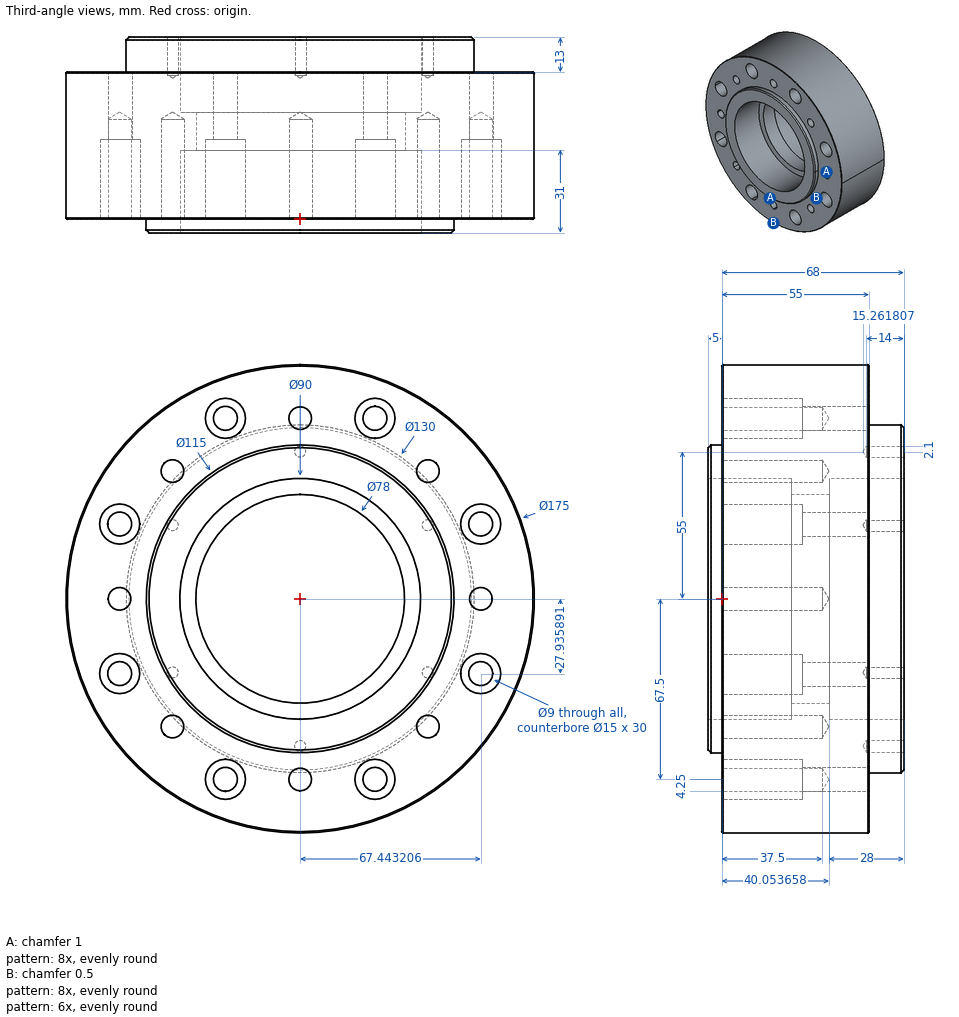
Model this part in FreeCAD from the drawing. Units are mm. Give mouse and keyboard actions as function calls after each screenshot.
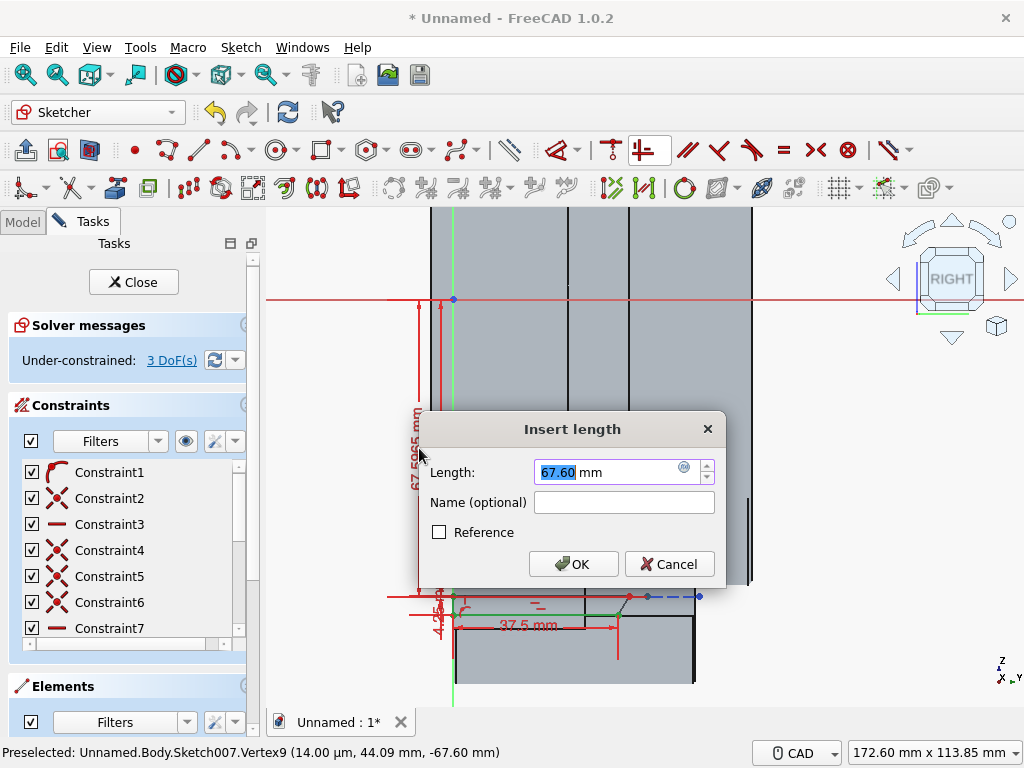
text(67.5)
key(Return)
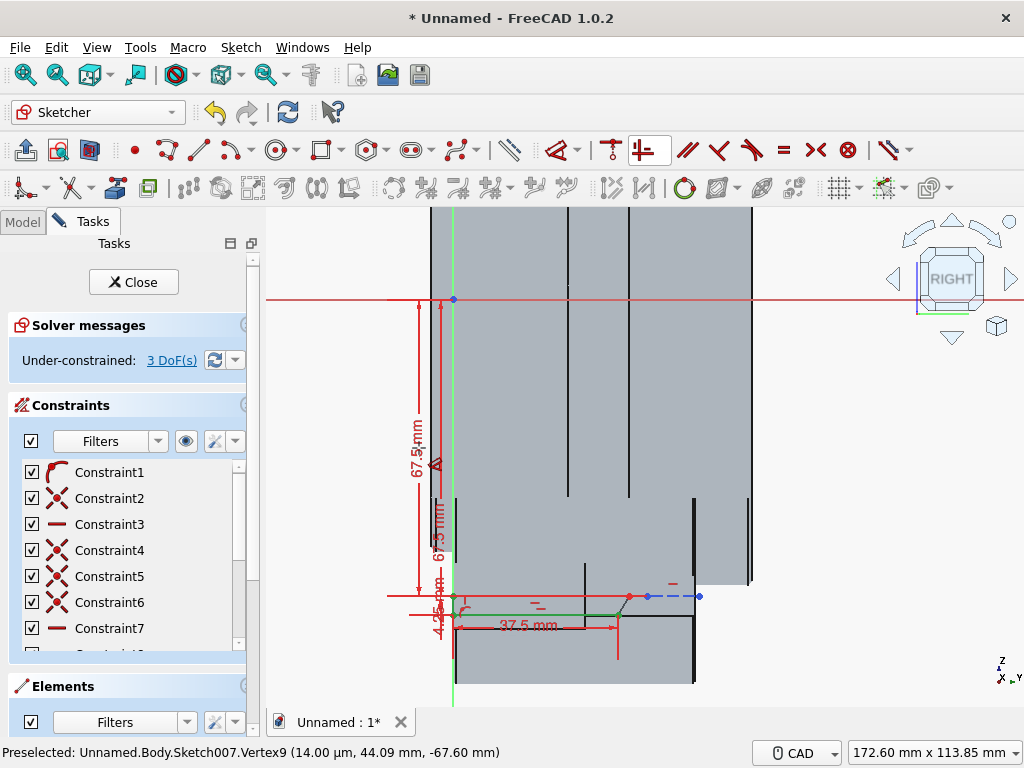
click(576, 596)
click(603, 630)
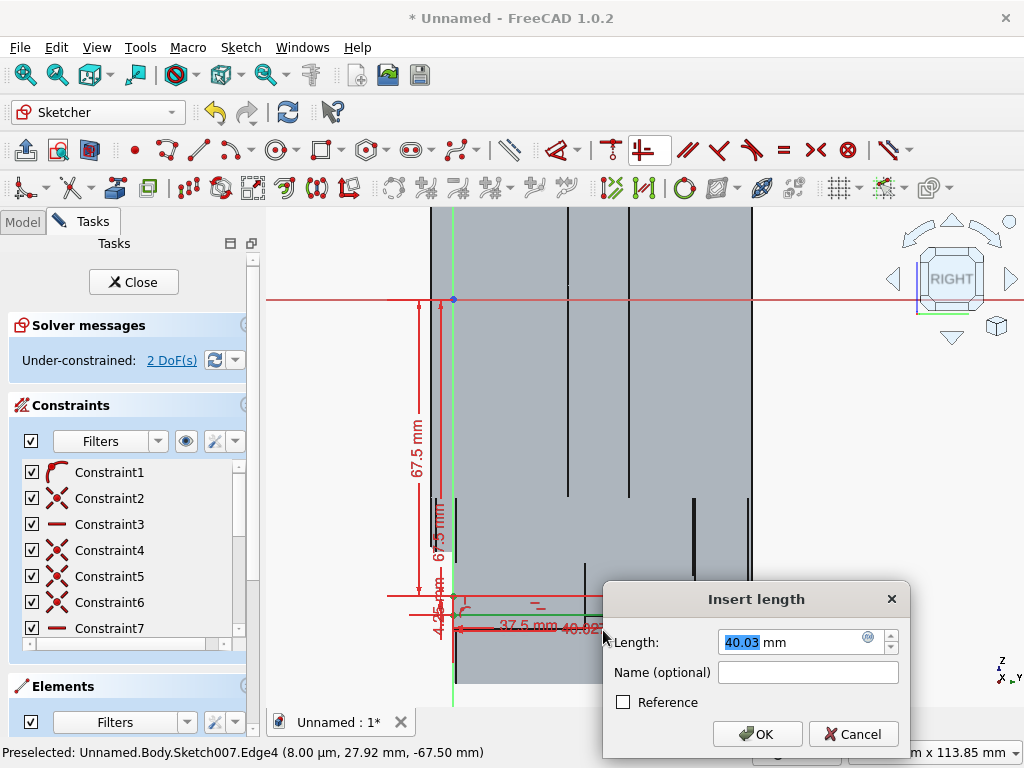
text(40.053658)
key(Return)
key(Escape)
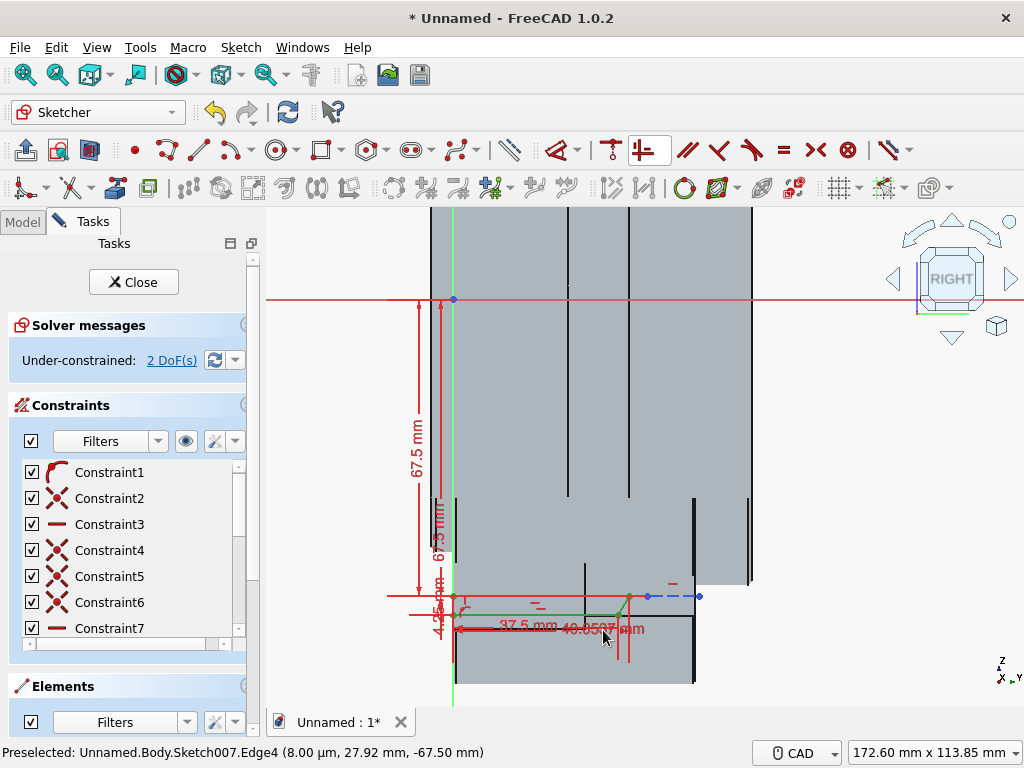
click(134, 282)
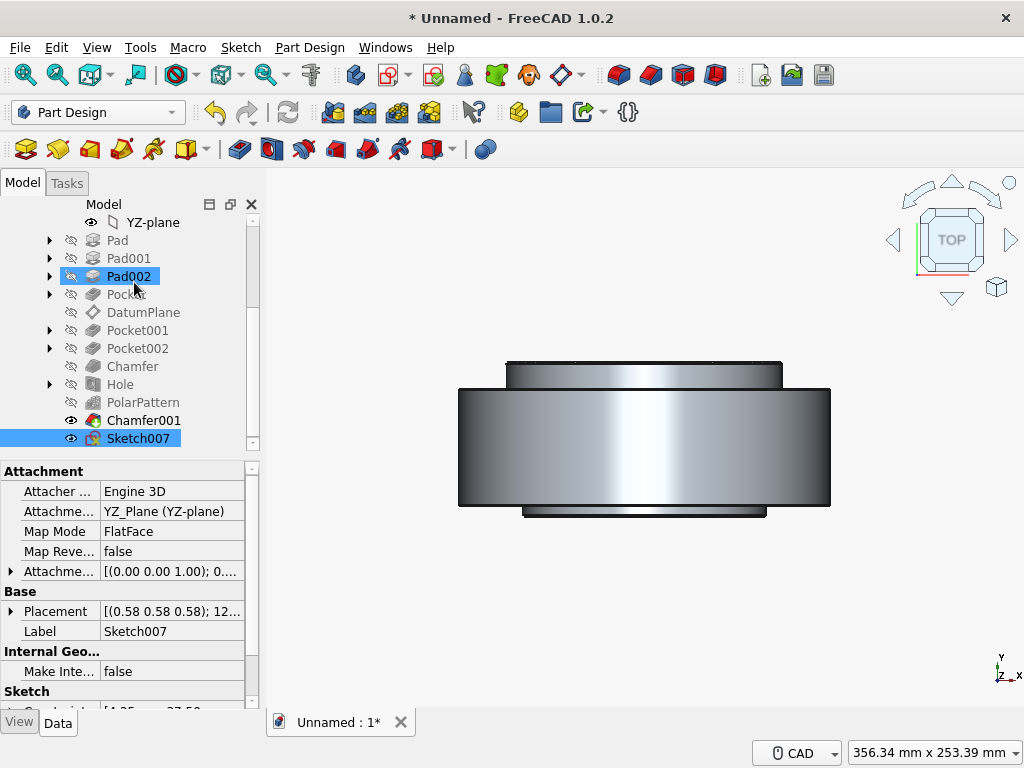
click(304, 150)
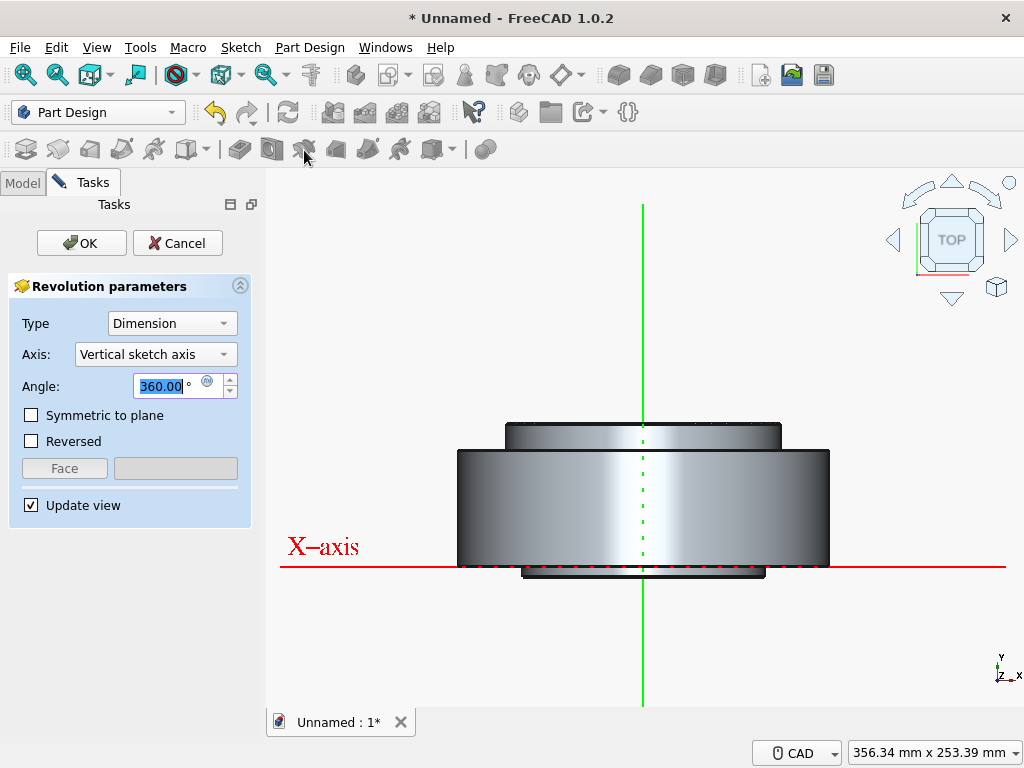
click(156, 354)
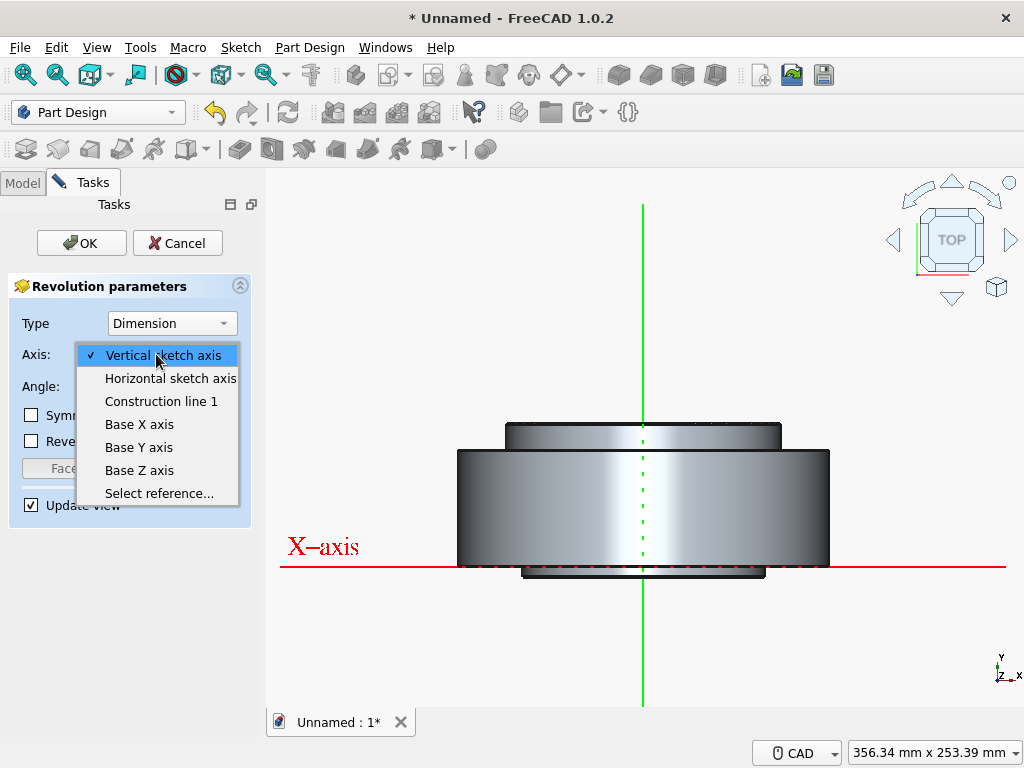
click(156, 402)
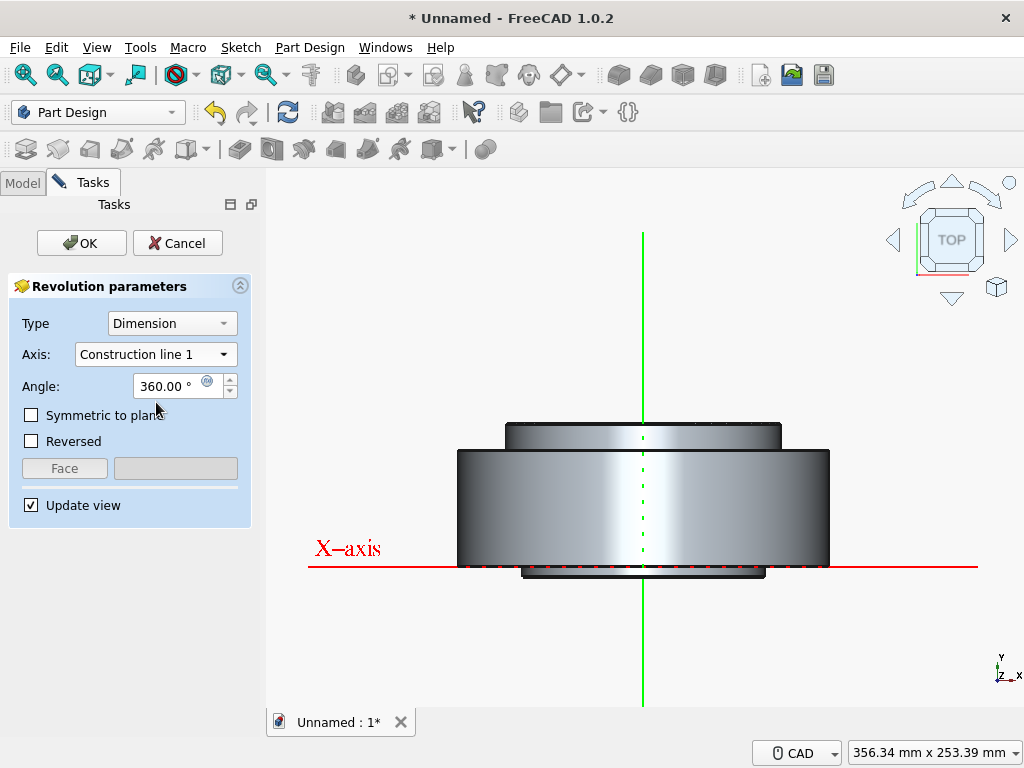
click(82, 243)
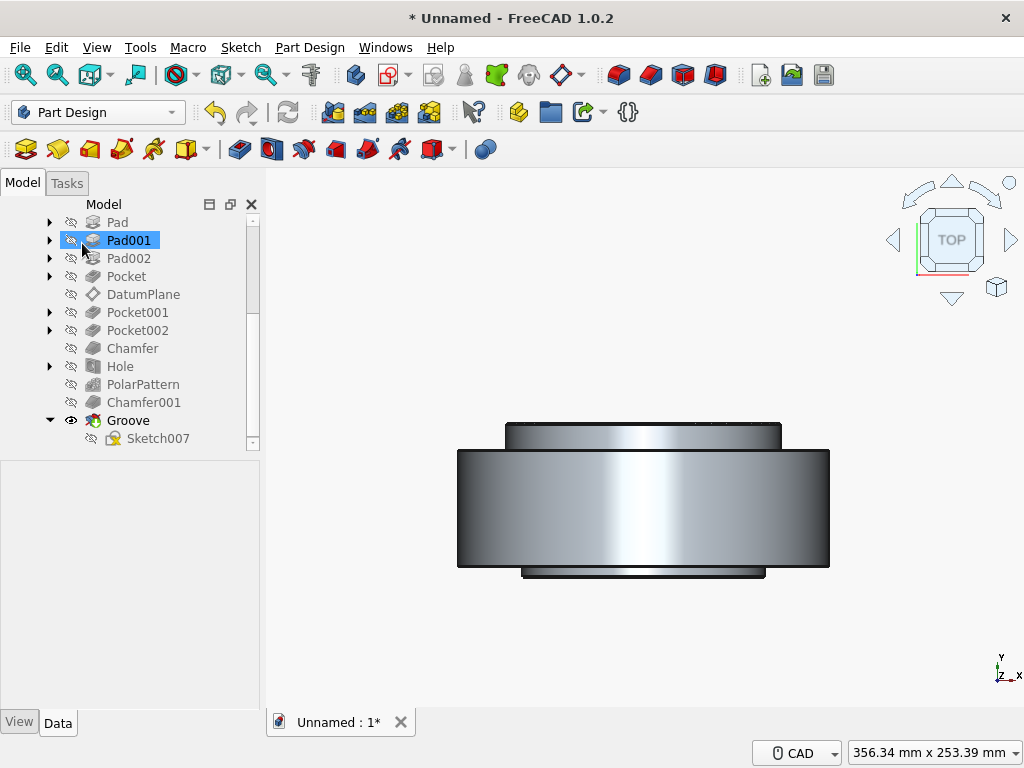
click(116, 420)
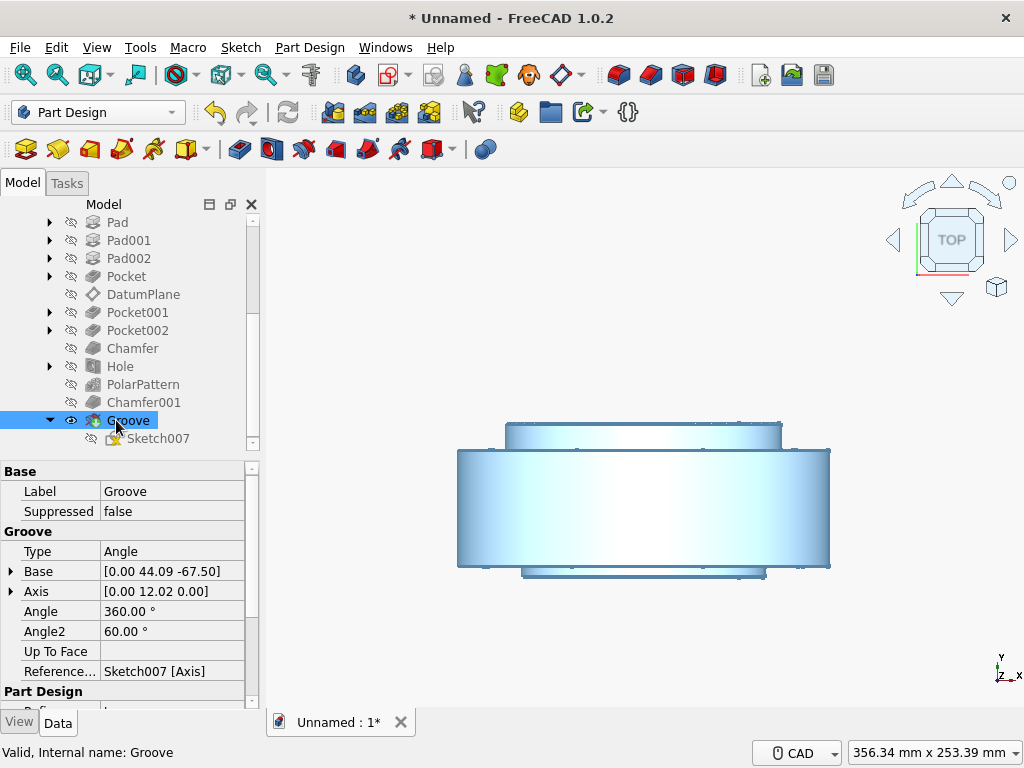
click(398, 112)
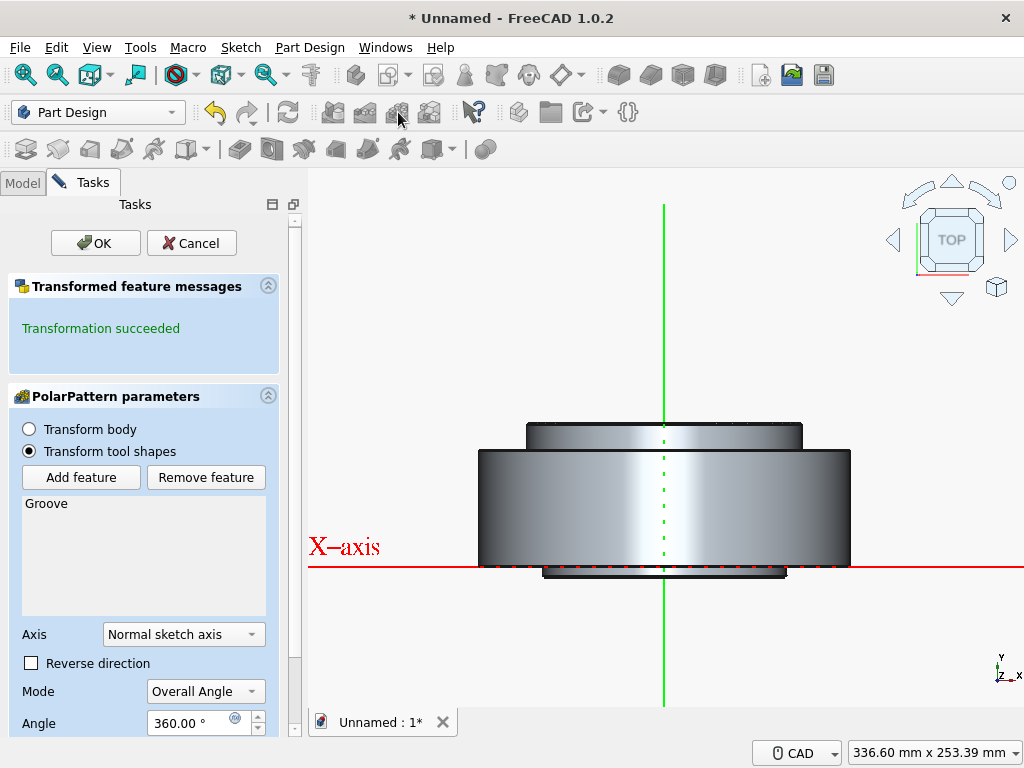
click(184, 634)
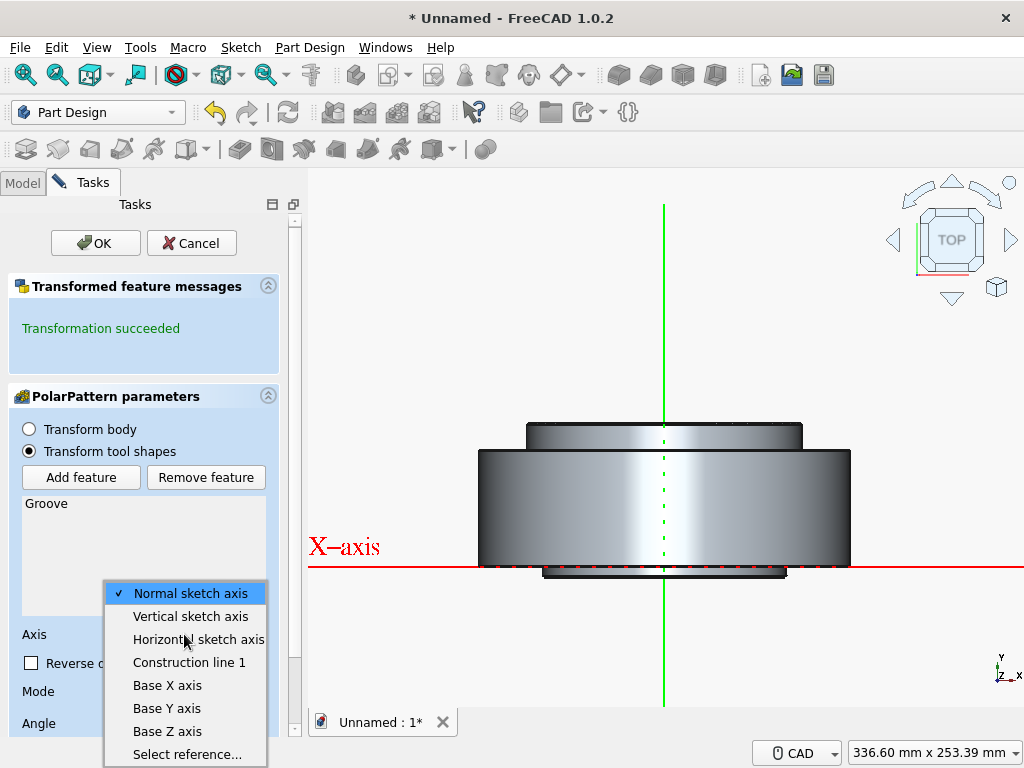
click(184, 708)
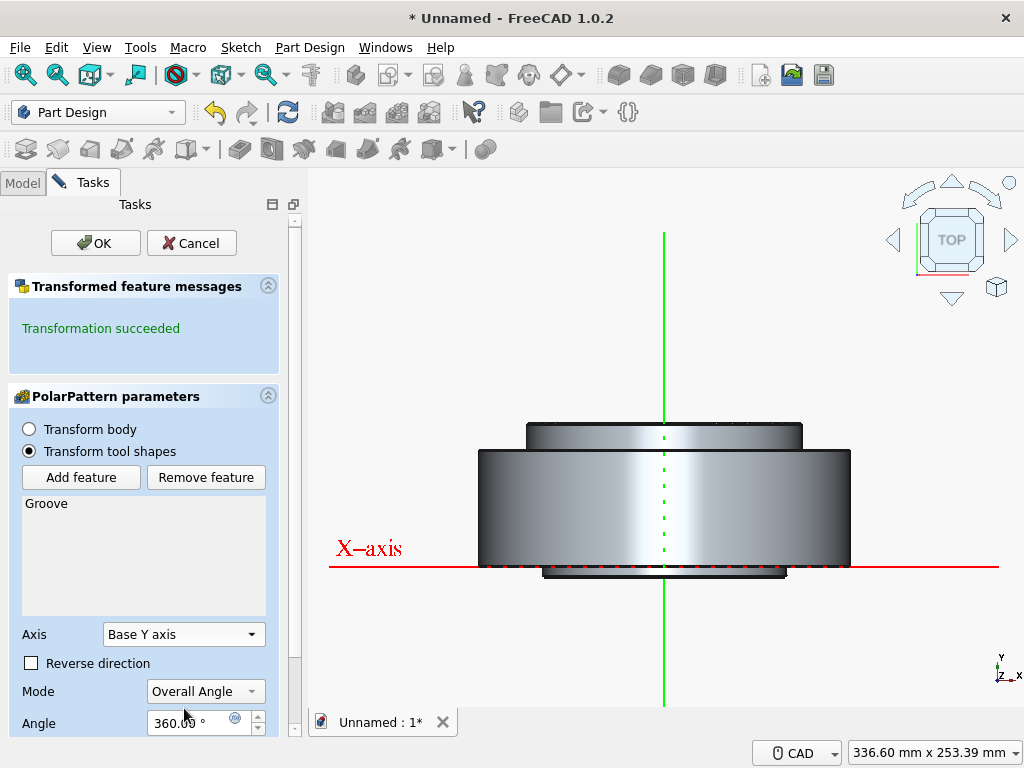
scroll(295, 475, down, 2)